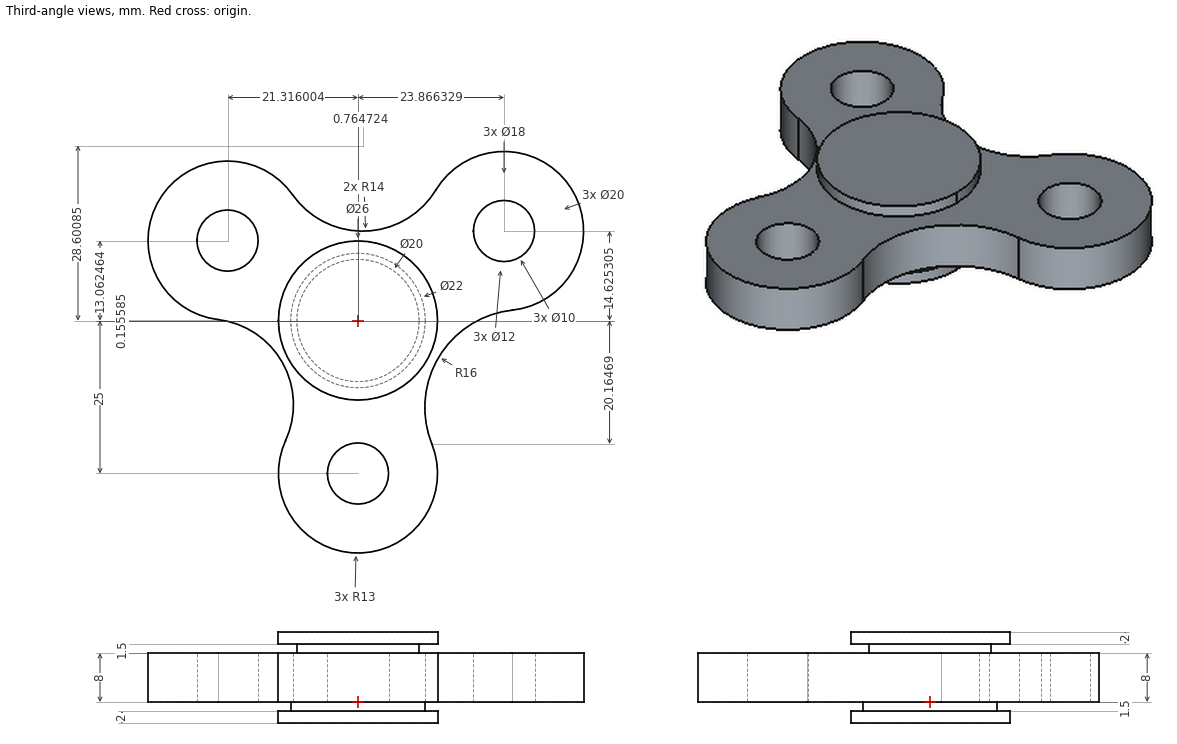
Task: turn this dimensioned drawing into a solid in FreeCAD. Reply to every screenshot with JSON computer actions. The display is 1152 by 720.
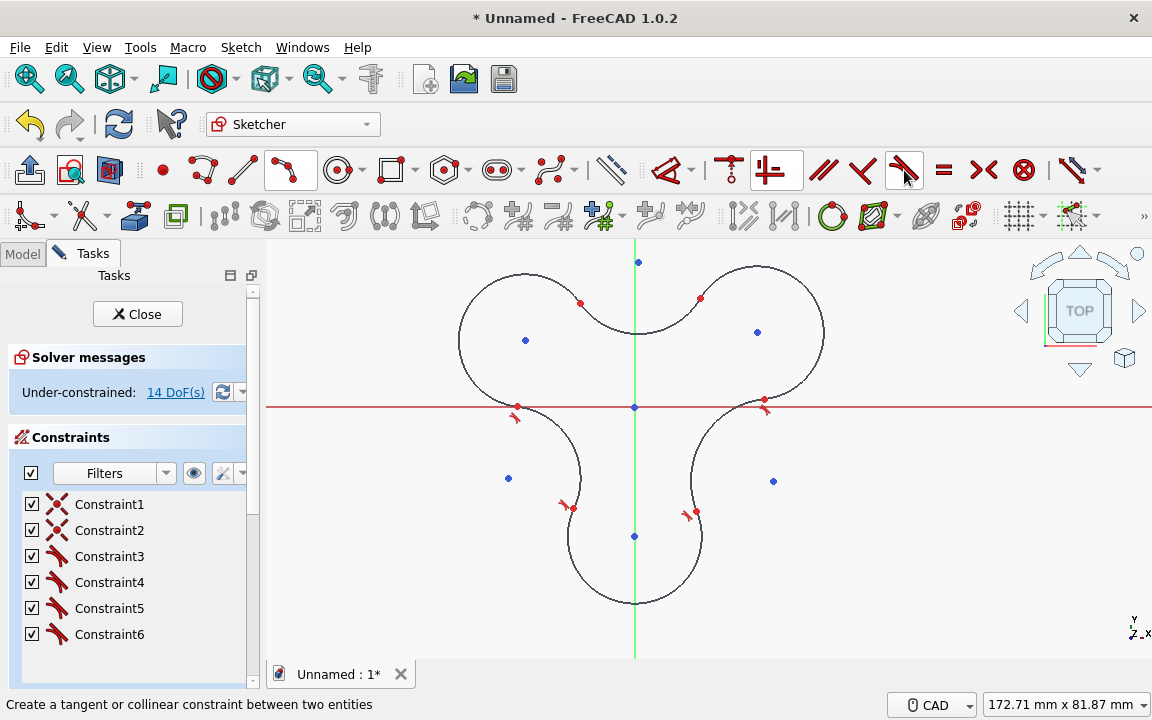
{"action": "left_click", "coordinate": [822, 349]}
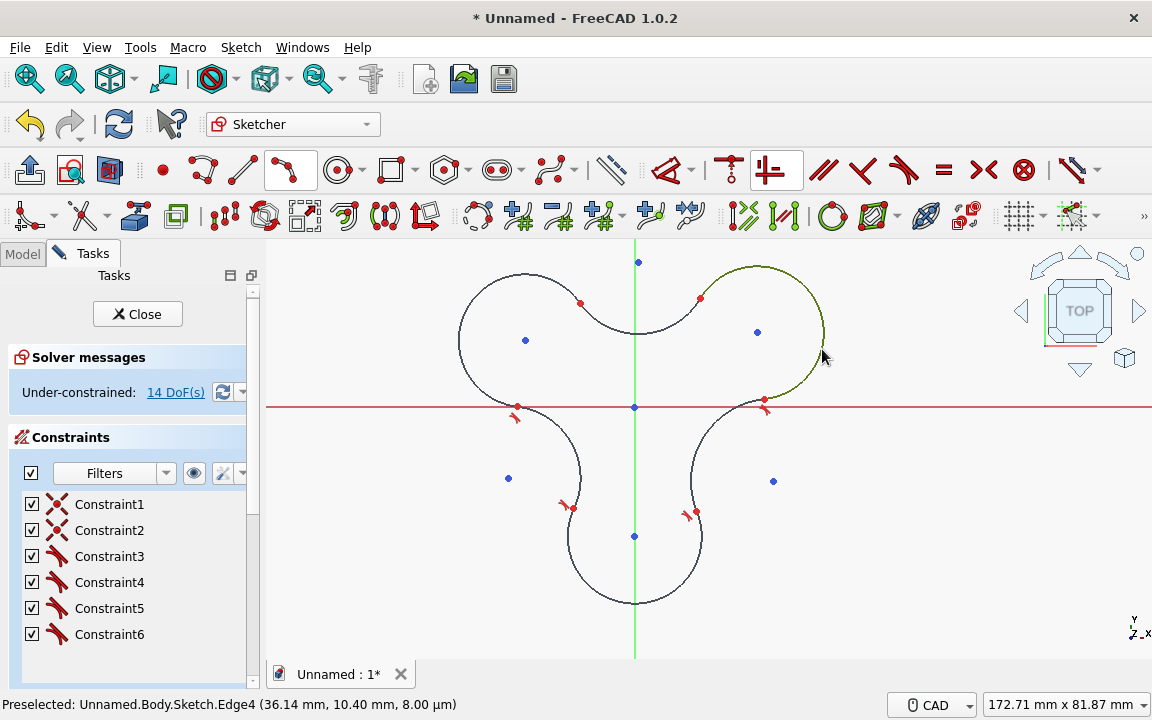
{"action": "left_click", "coordinate": [614, 329]}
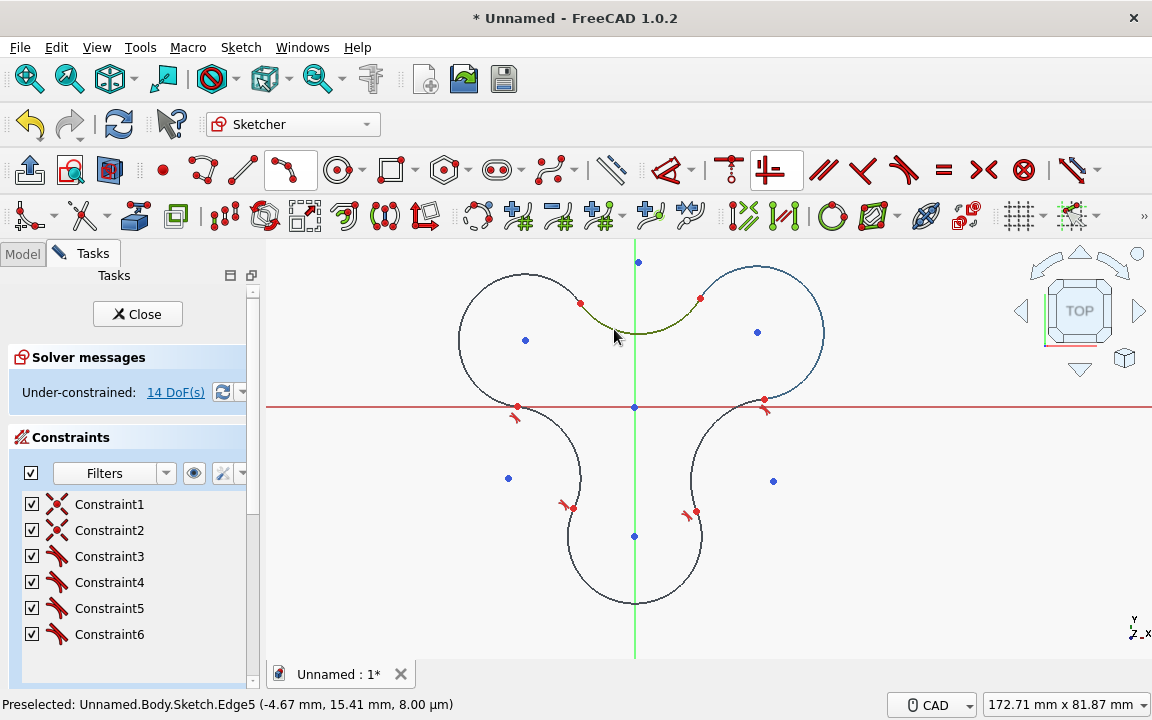
{"action": "left_click", "coordinate": [904, 170]}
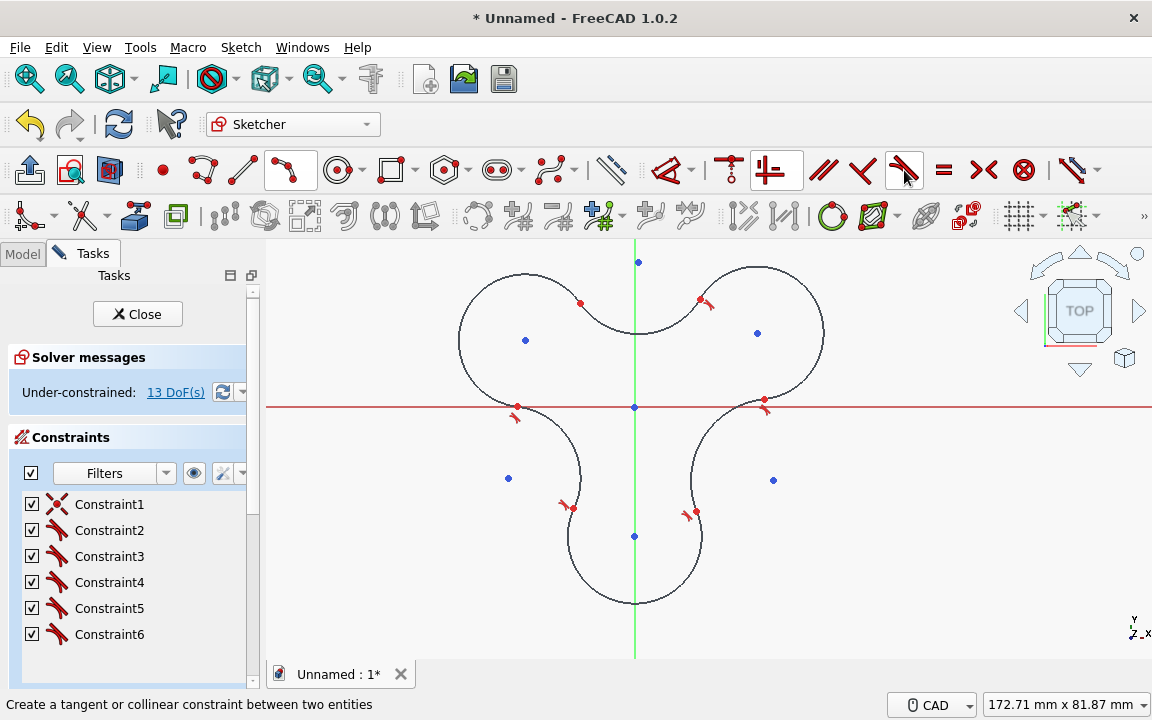
{"action": "left_click", "coordinate": [614, 329]}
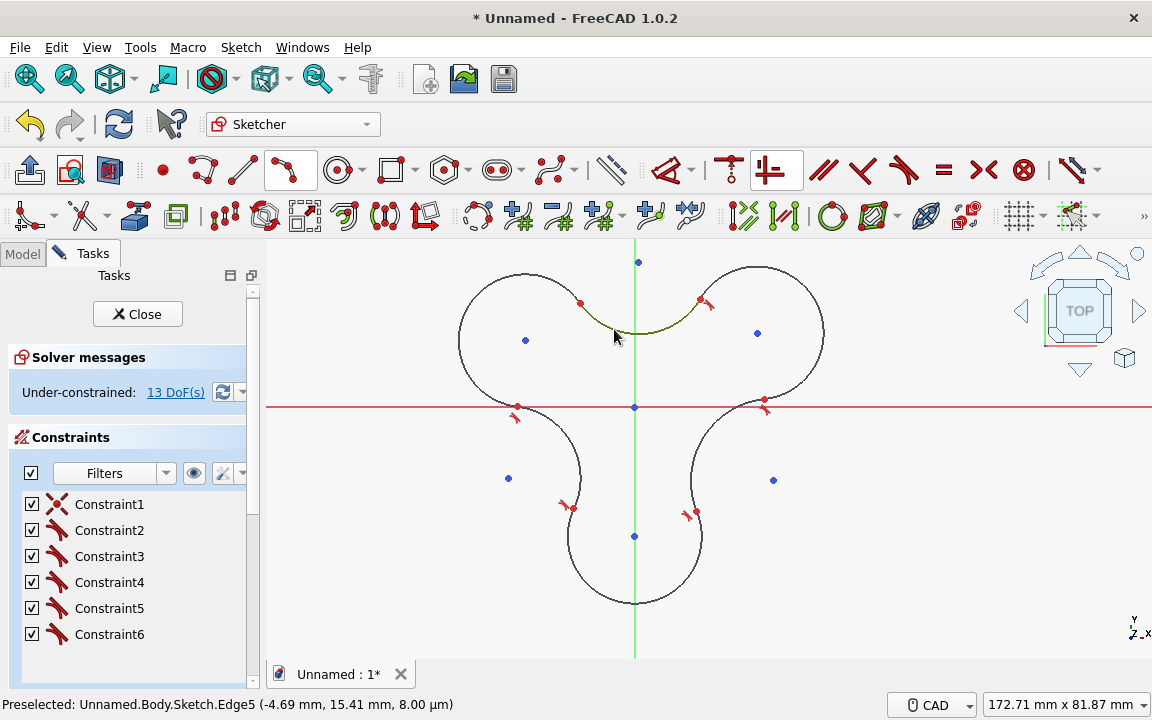
{"action": "left_click", "coordinate": [511, 276]}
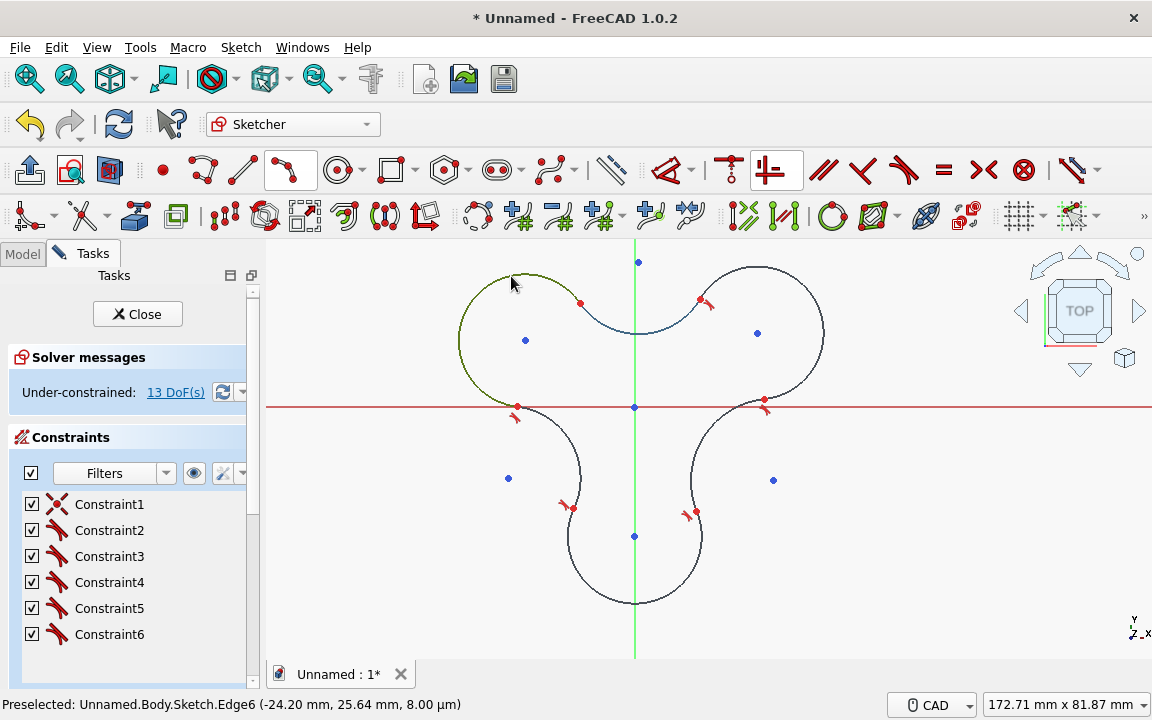
{"action": "left_click", "coordinate": [904, 170]}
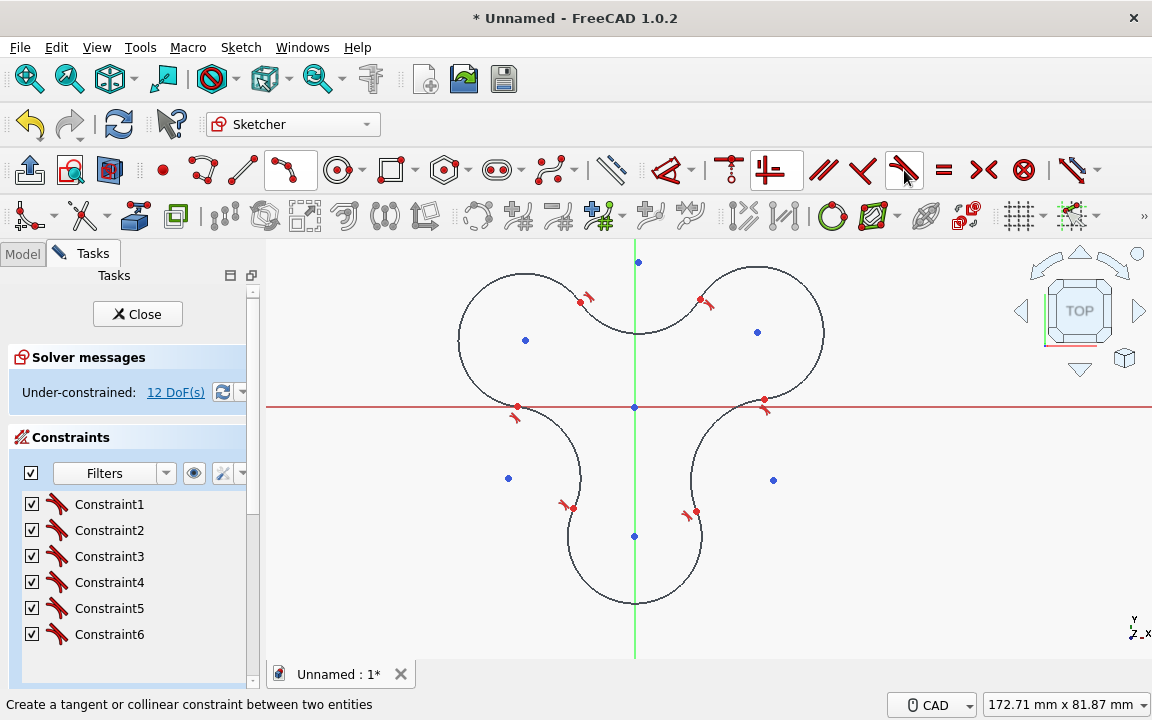
{"action": "left_click", "coordinate": [586, 582]}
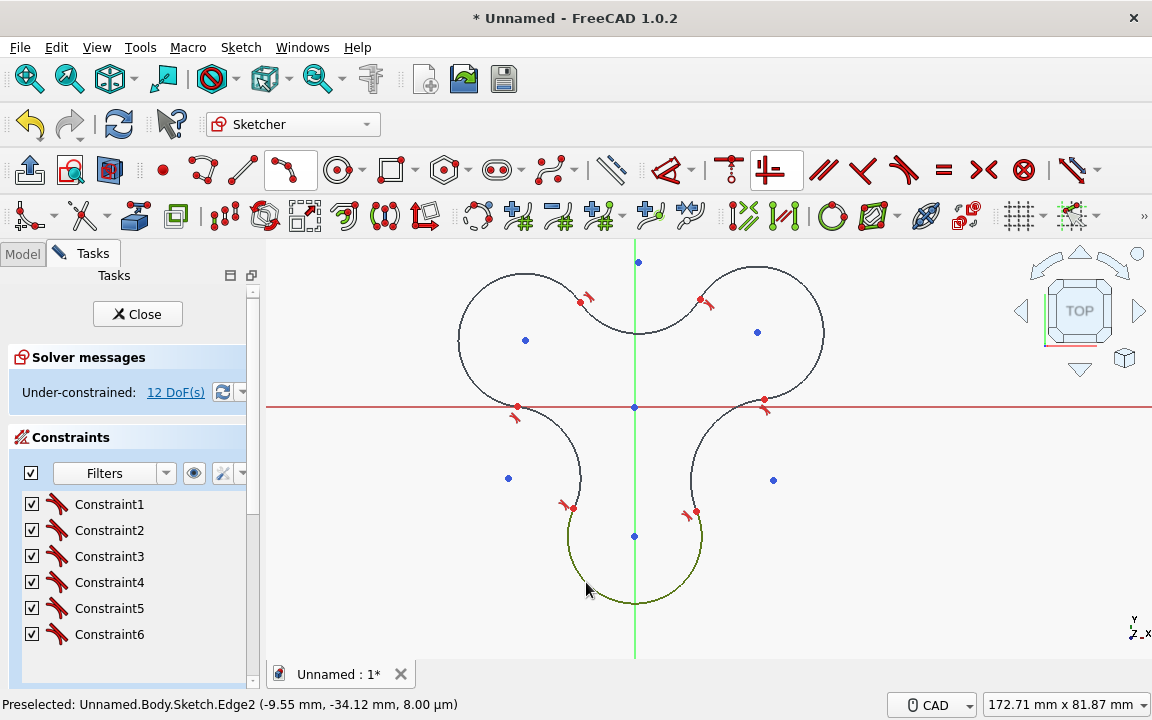
{"action": "left_click", "coordinate": [822, 349]}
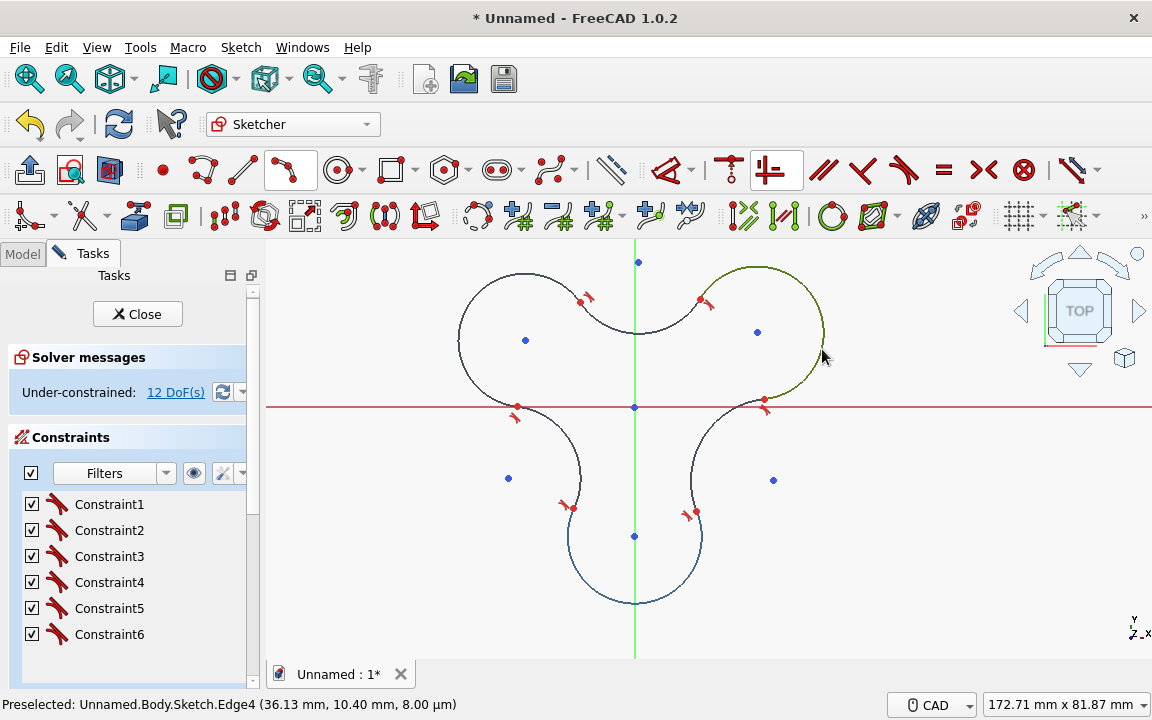
{"action": "left_click", "coordinate": [510, 275]}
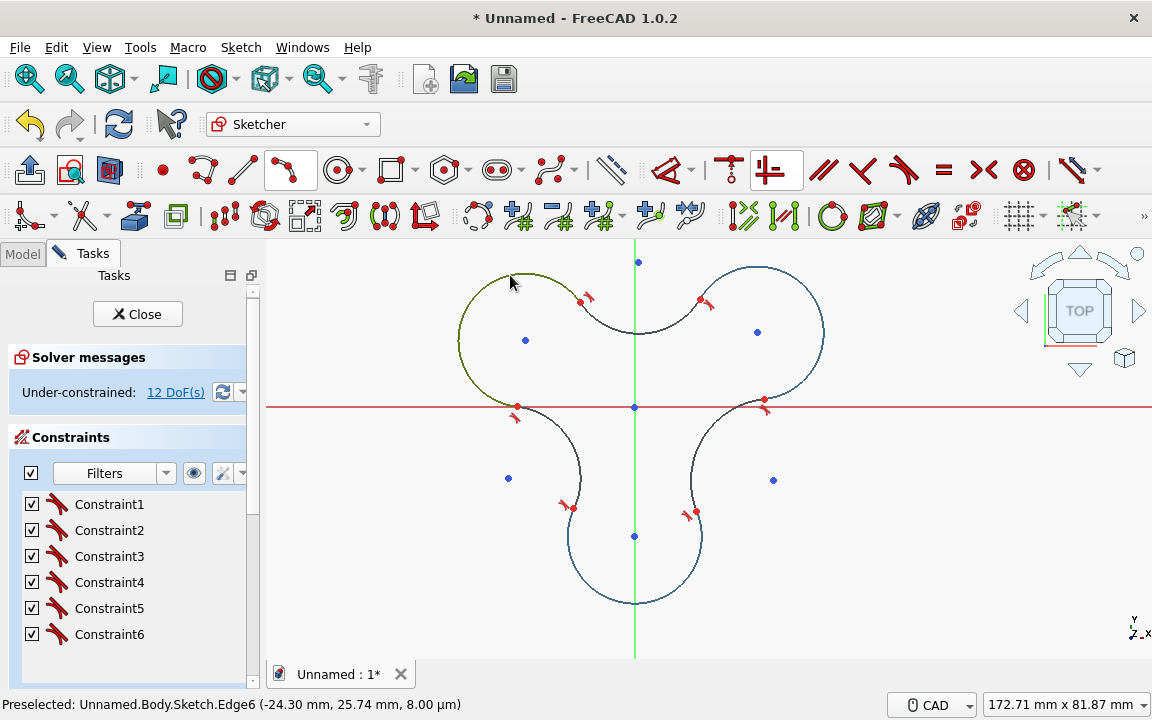
{"action": "left_click", "coordinate": [944, 170]}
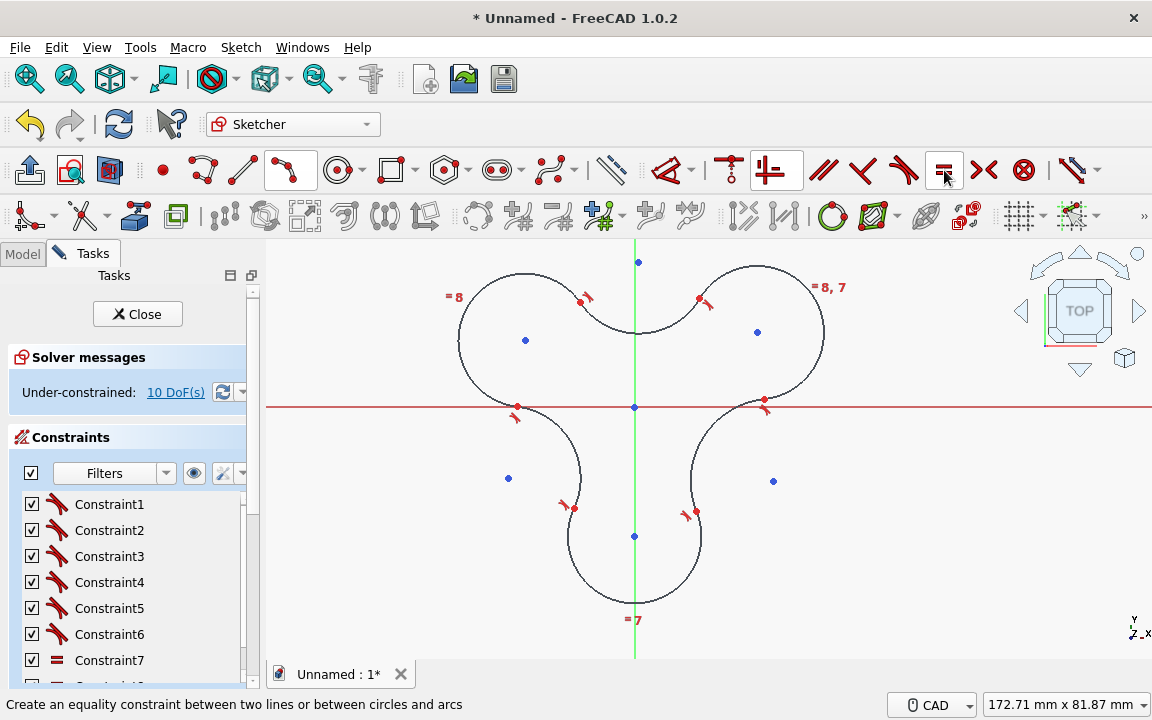
{"action": "left_click", "coordinate": [580, 469]}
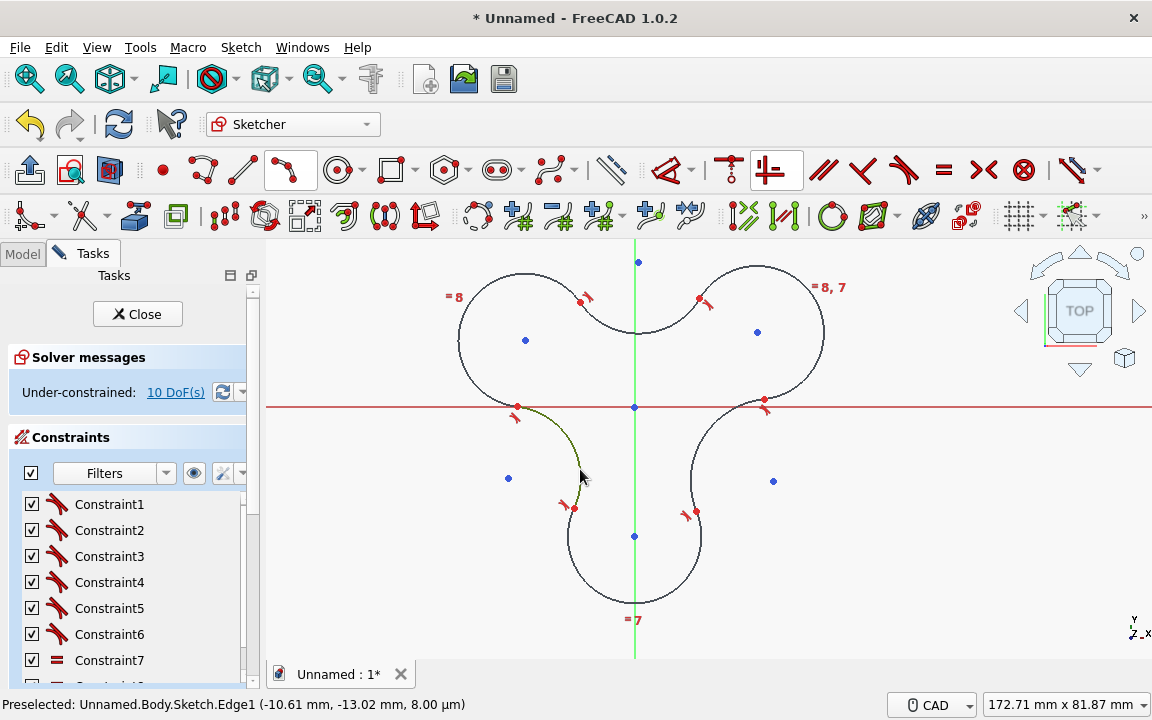
{"action": "left_click", "coordinate": [613, 329]}